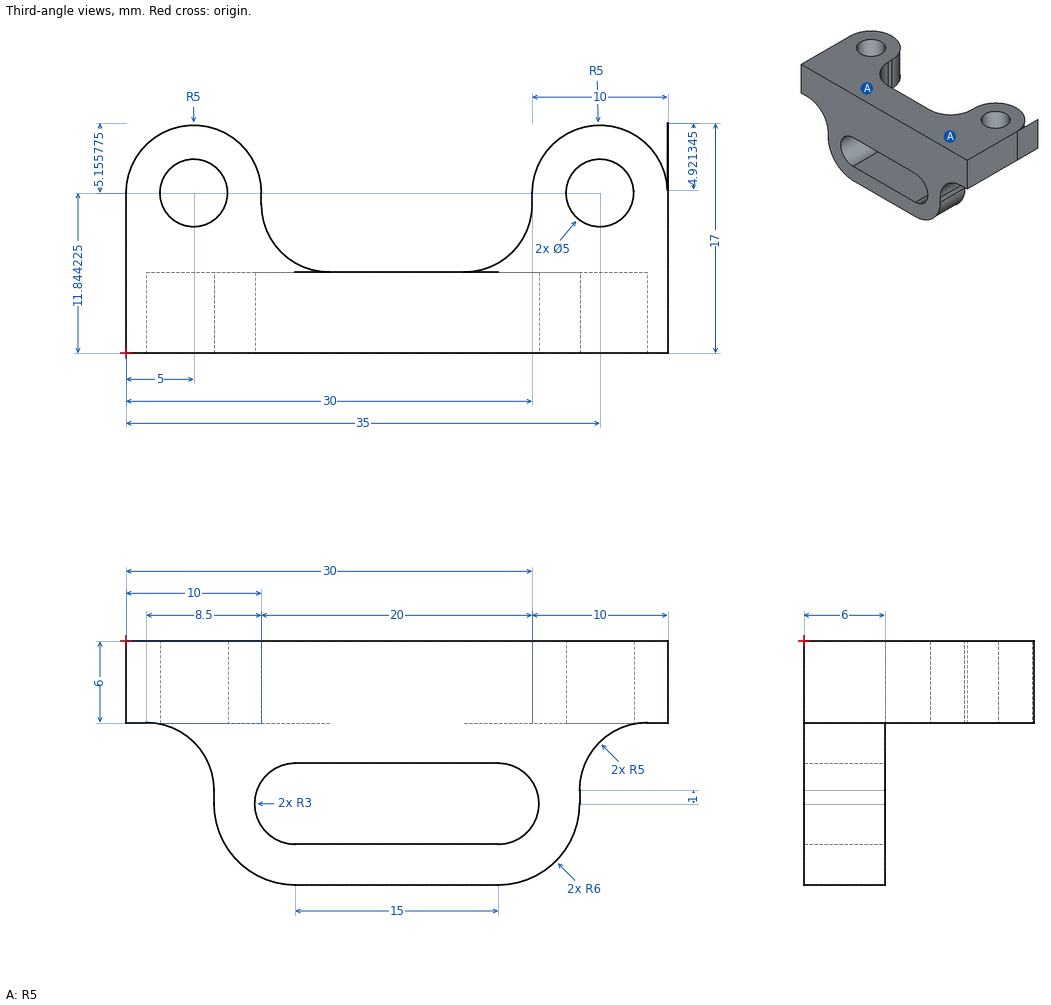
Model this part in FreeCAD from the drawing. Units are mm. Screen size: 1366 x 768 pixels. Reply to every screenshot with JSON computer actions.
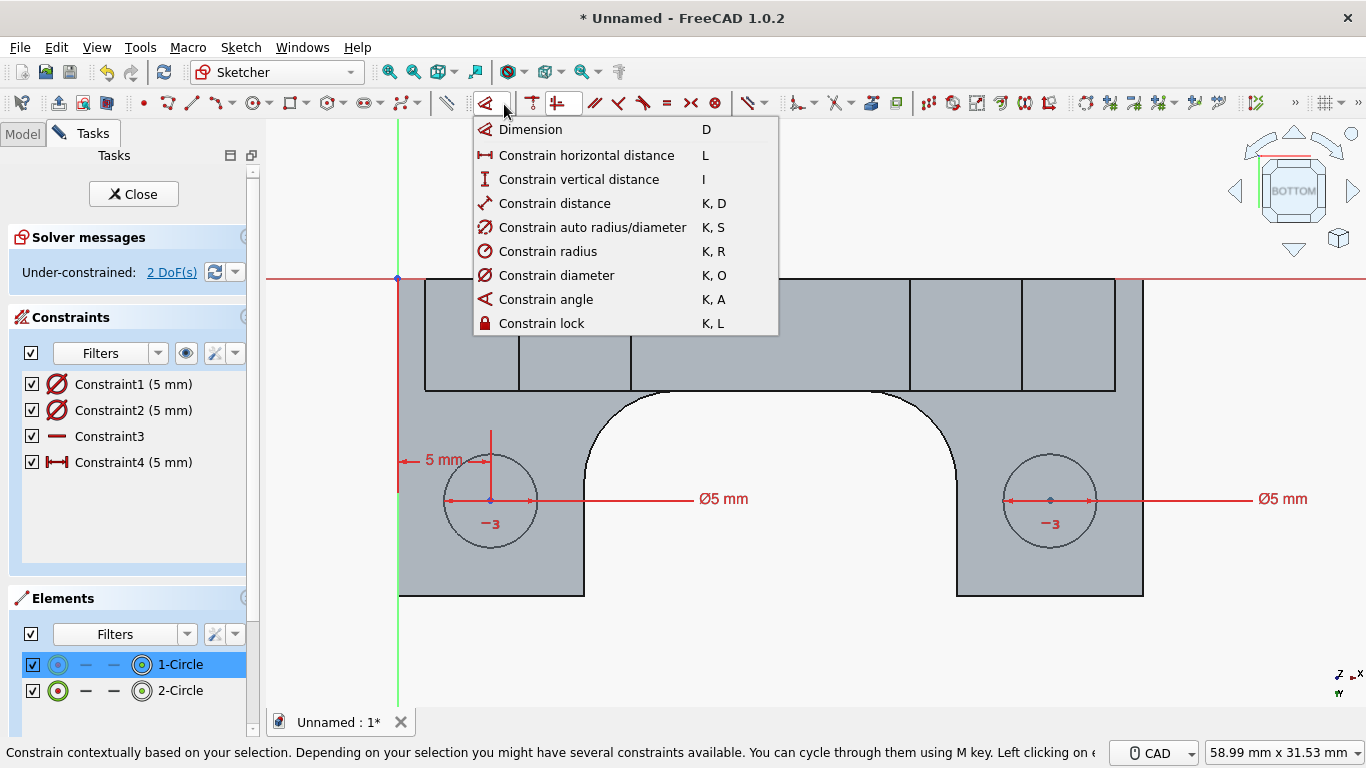
{"action": "left_click", "coordinate": [626, 155]}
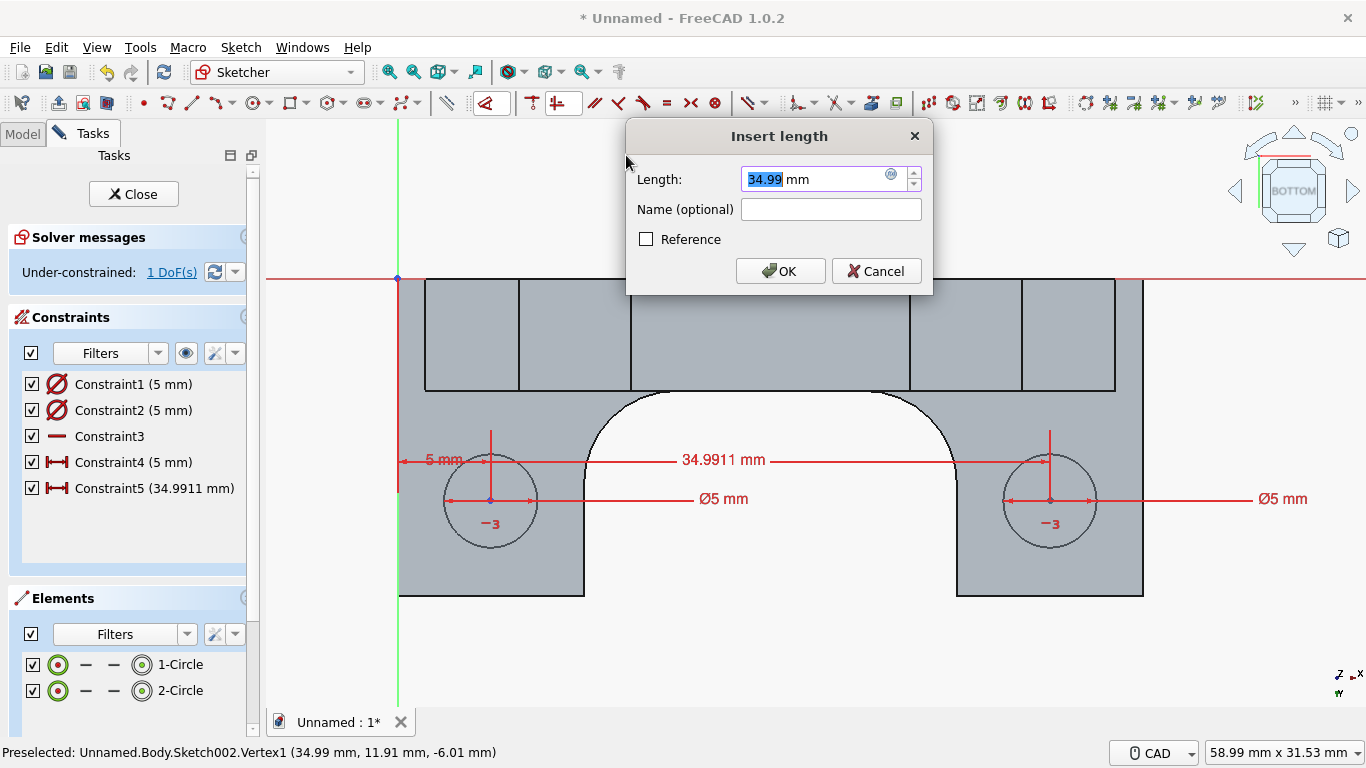
{"action": "type", "text": "35"}
{"action": "key", "text": "Return"}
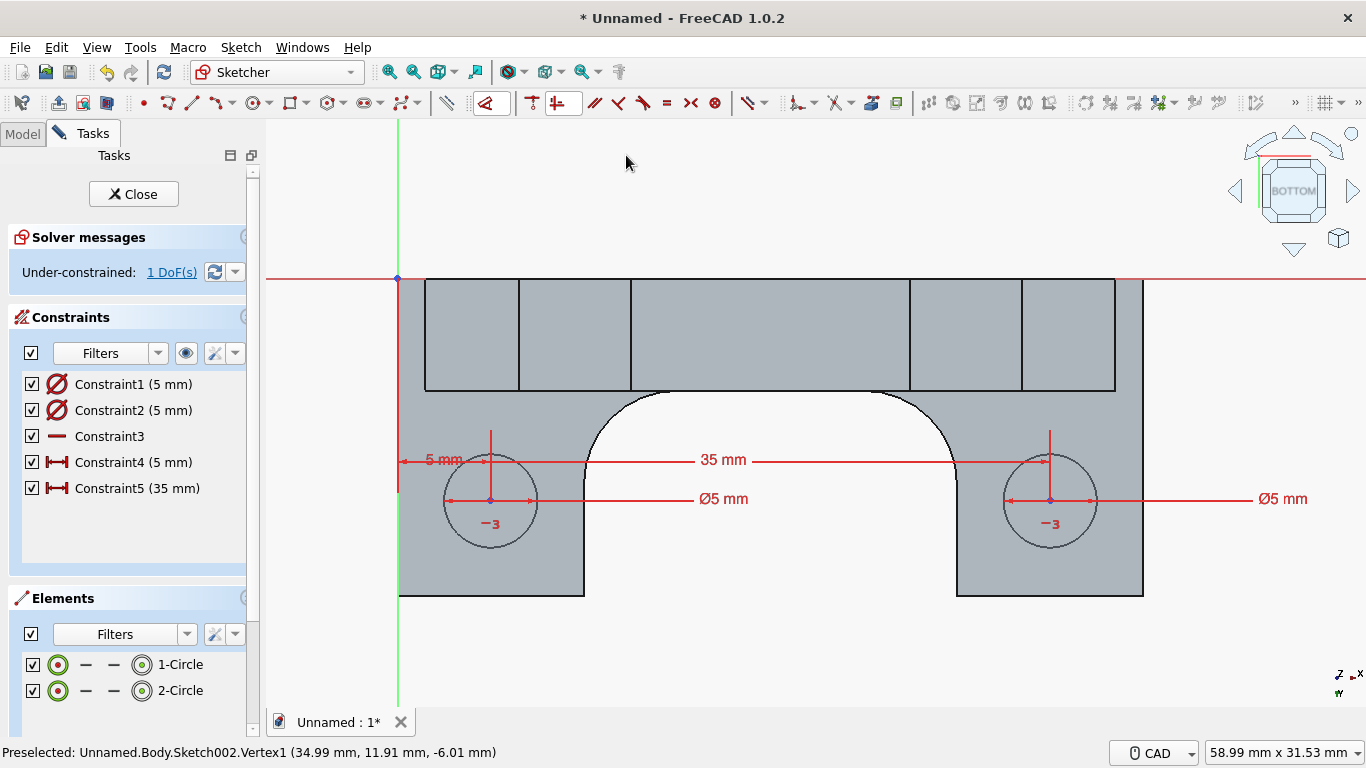
{"action": "left_click", "coordinate": [1050, 501]}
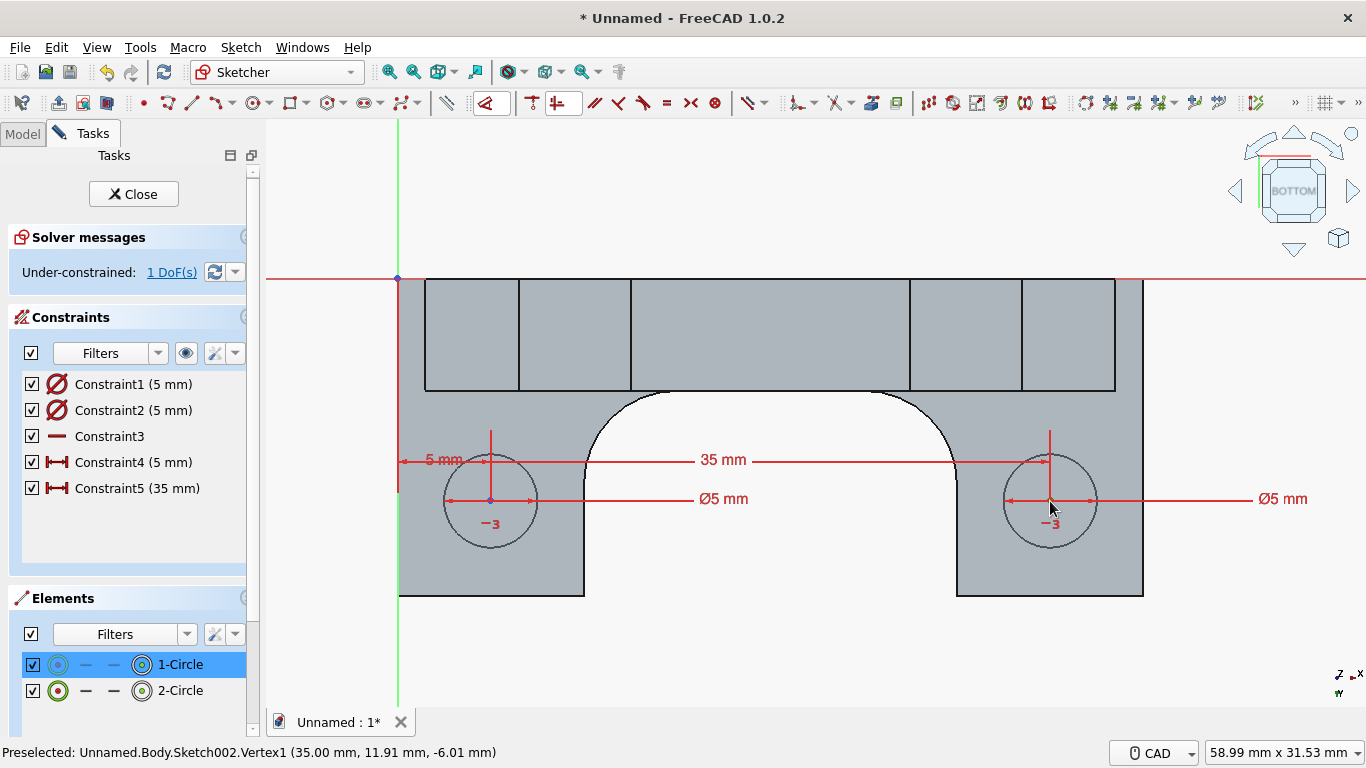
{"action": "key", "text": "i"}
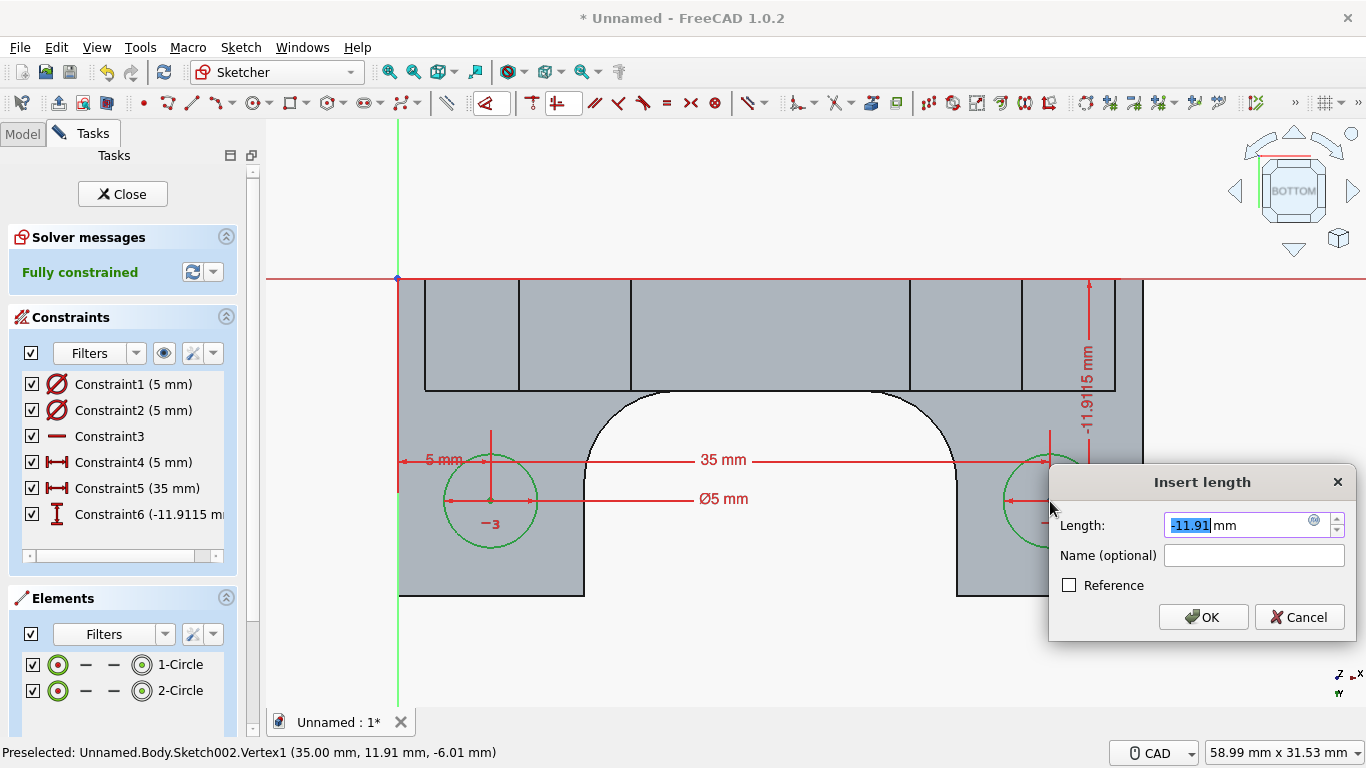
{"action": "type", "text": "-11.844225"}
{"action": "key", "text": "Return"}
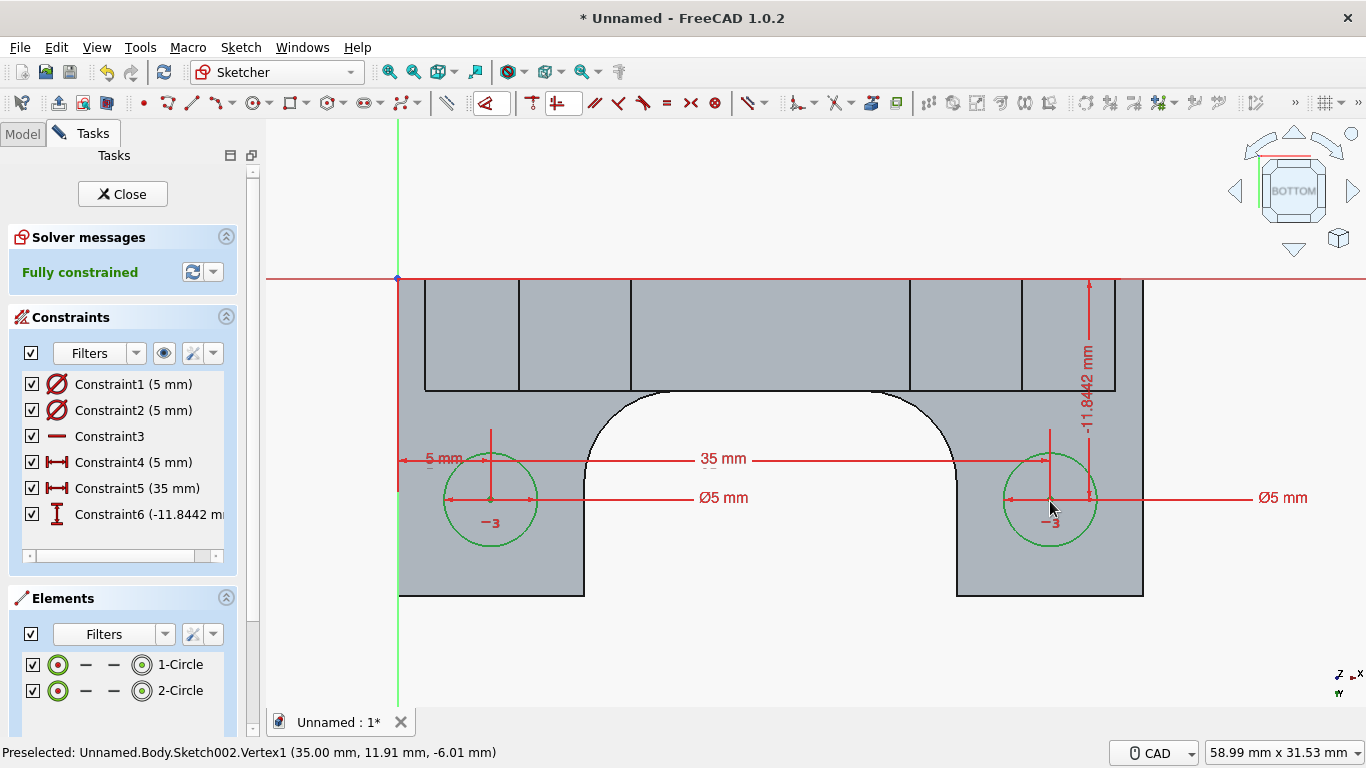
{"action": "left_click", "coordinate": [123, 194]}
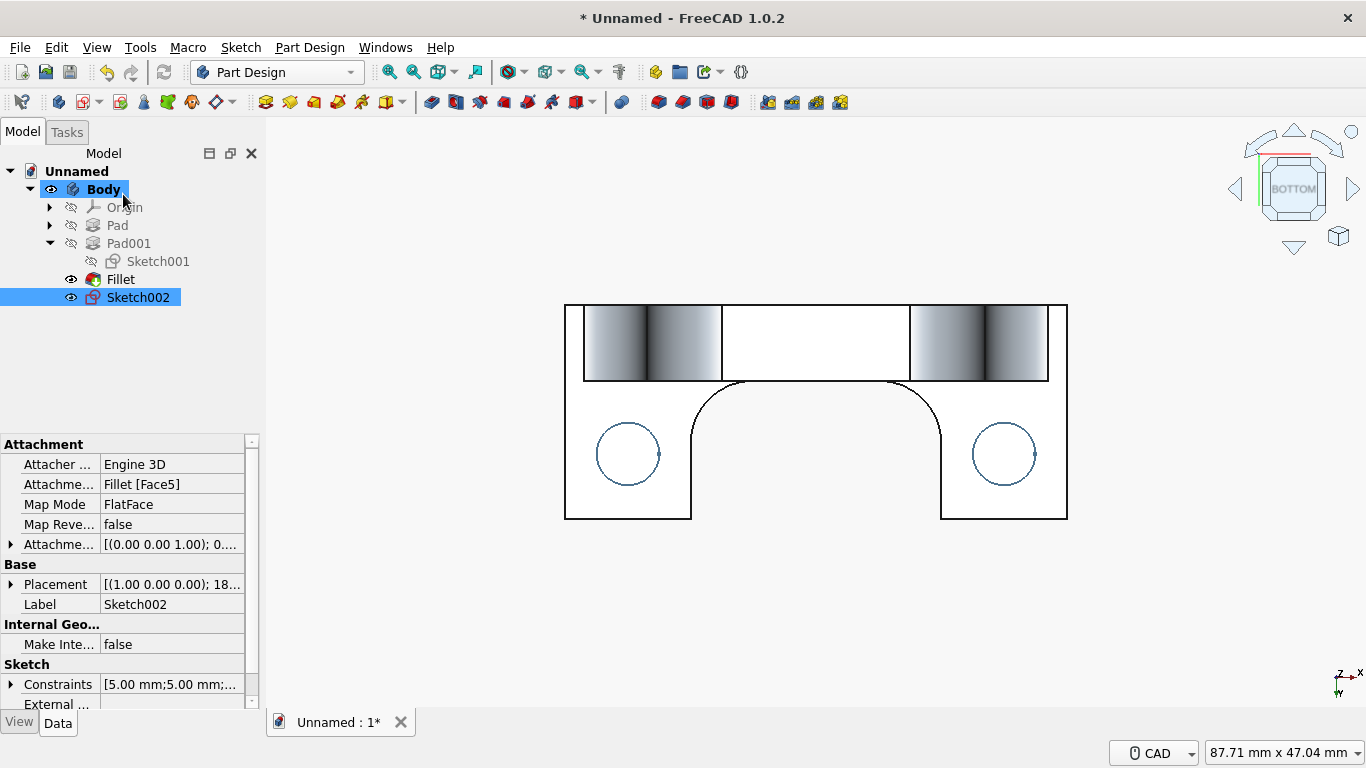
{"action": "left_click", "coordinate": [432, 102]}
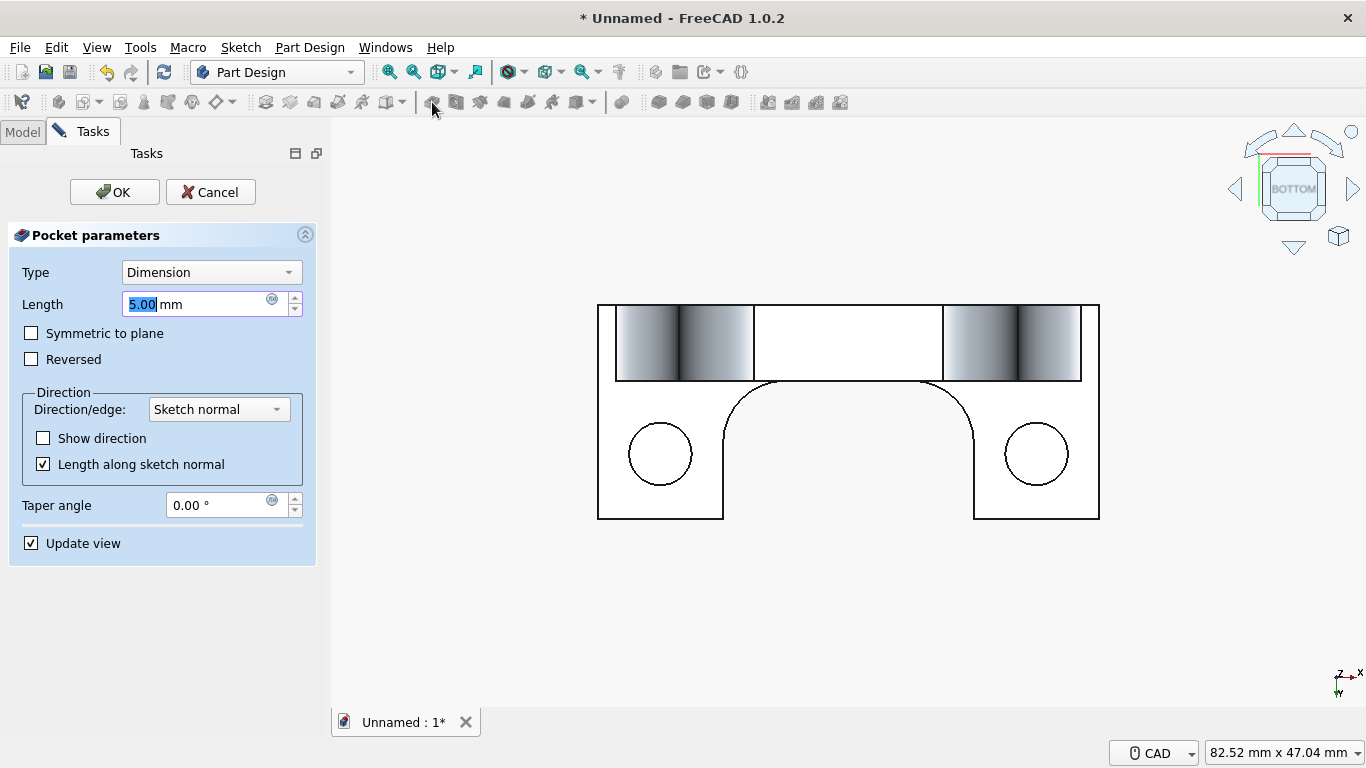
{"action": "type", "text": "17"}
{"action": "key", "text": "Tab"}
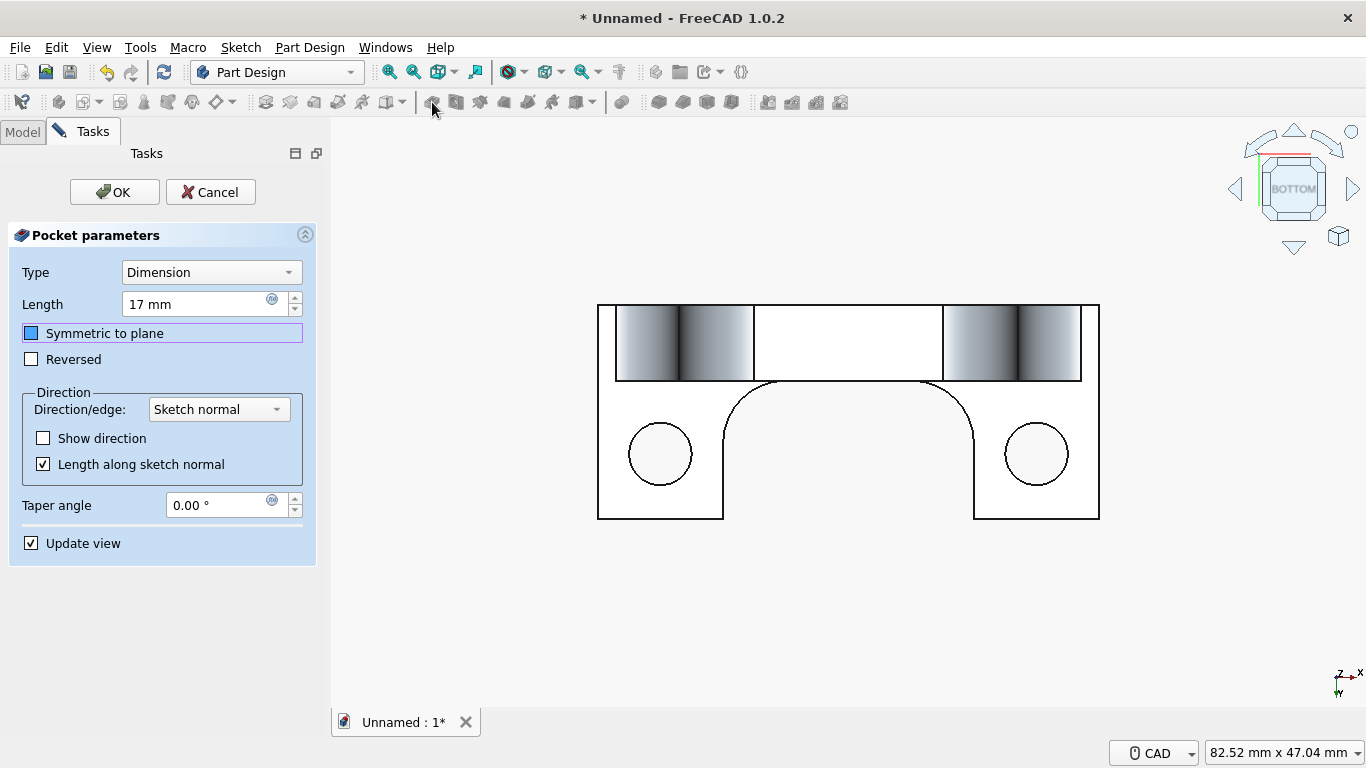
{"action": "left_click", "coordinate": [115, 192]}